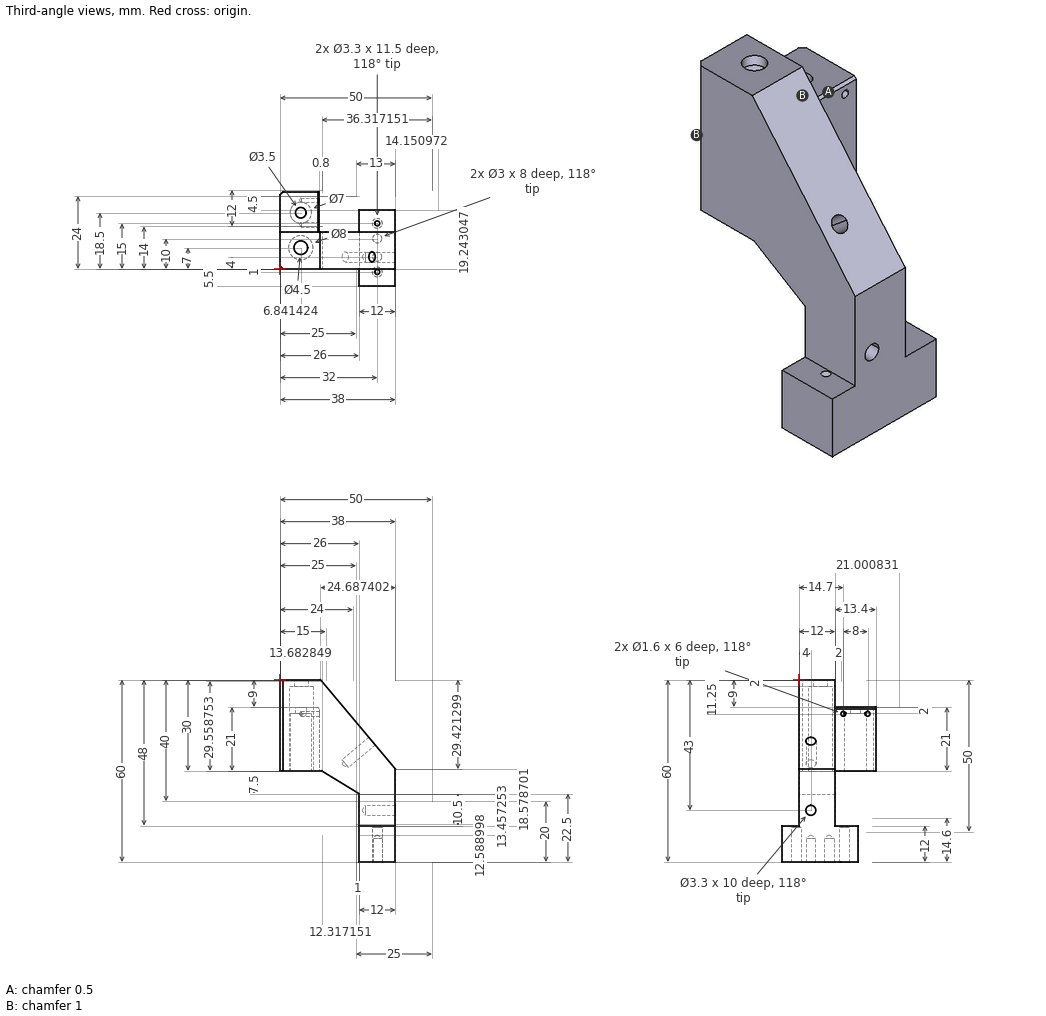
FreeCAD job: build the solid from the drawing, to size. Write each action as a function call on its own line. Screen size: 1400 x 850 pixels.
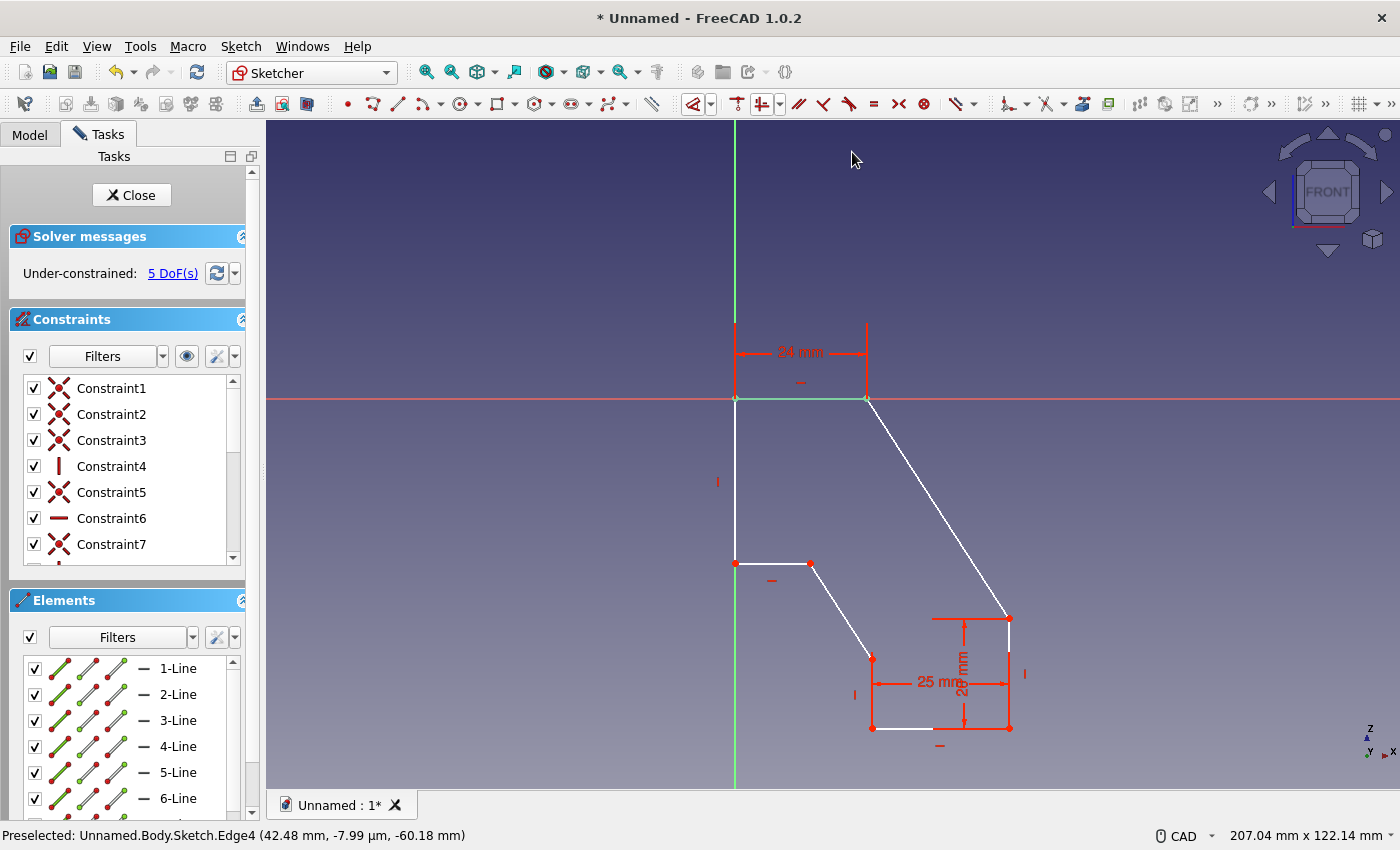
click(735, 514)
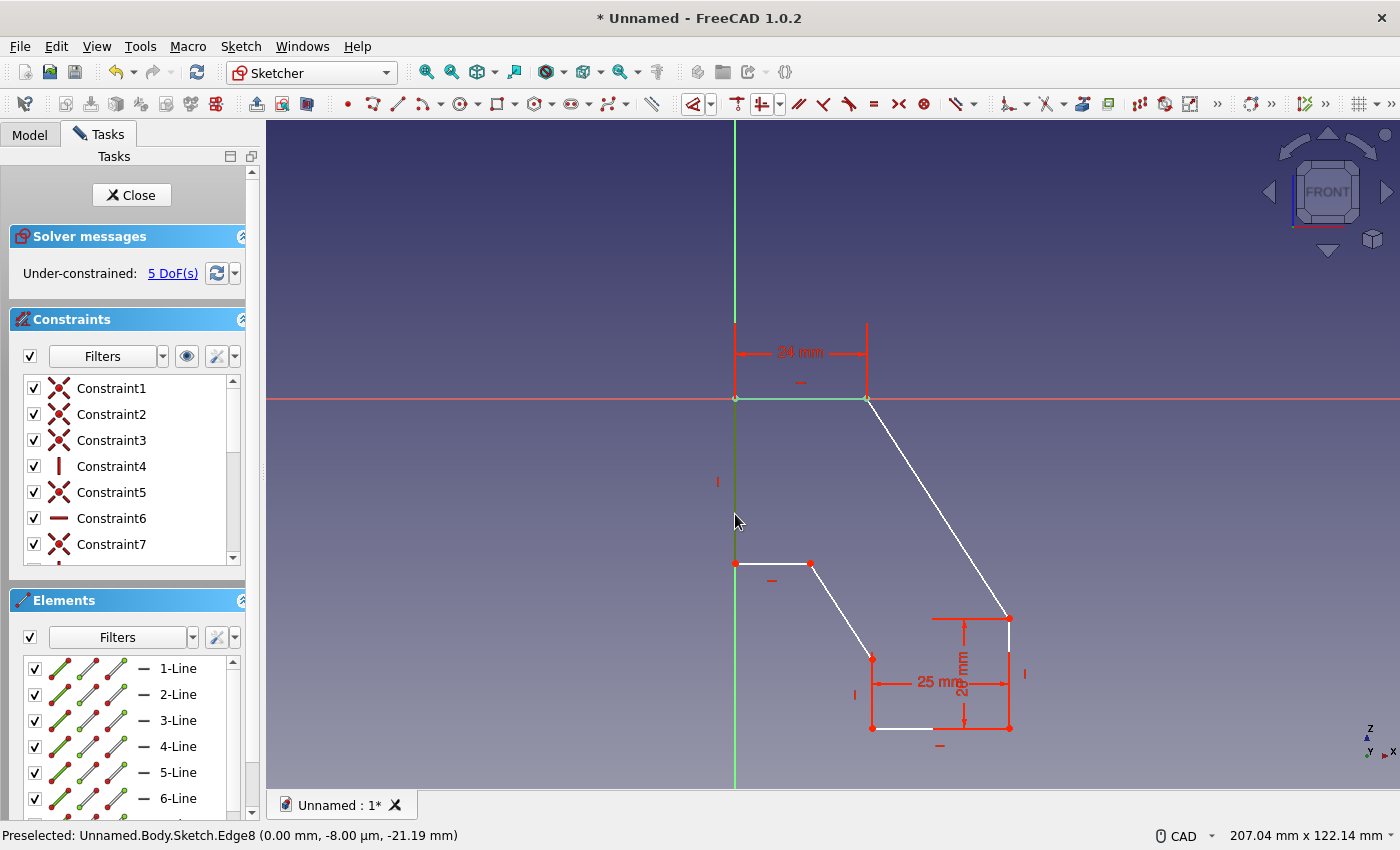
key(i)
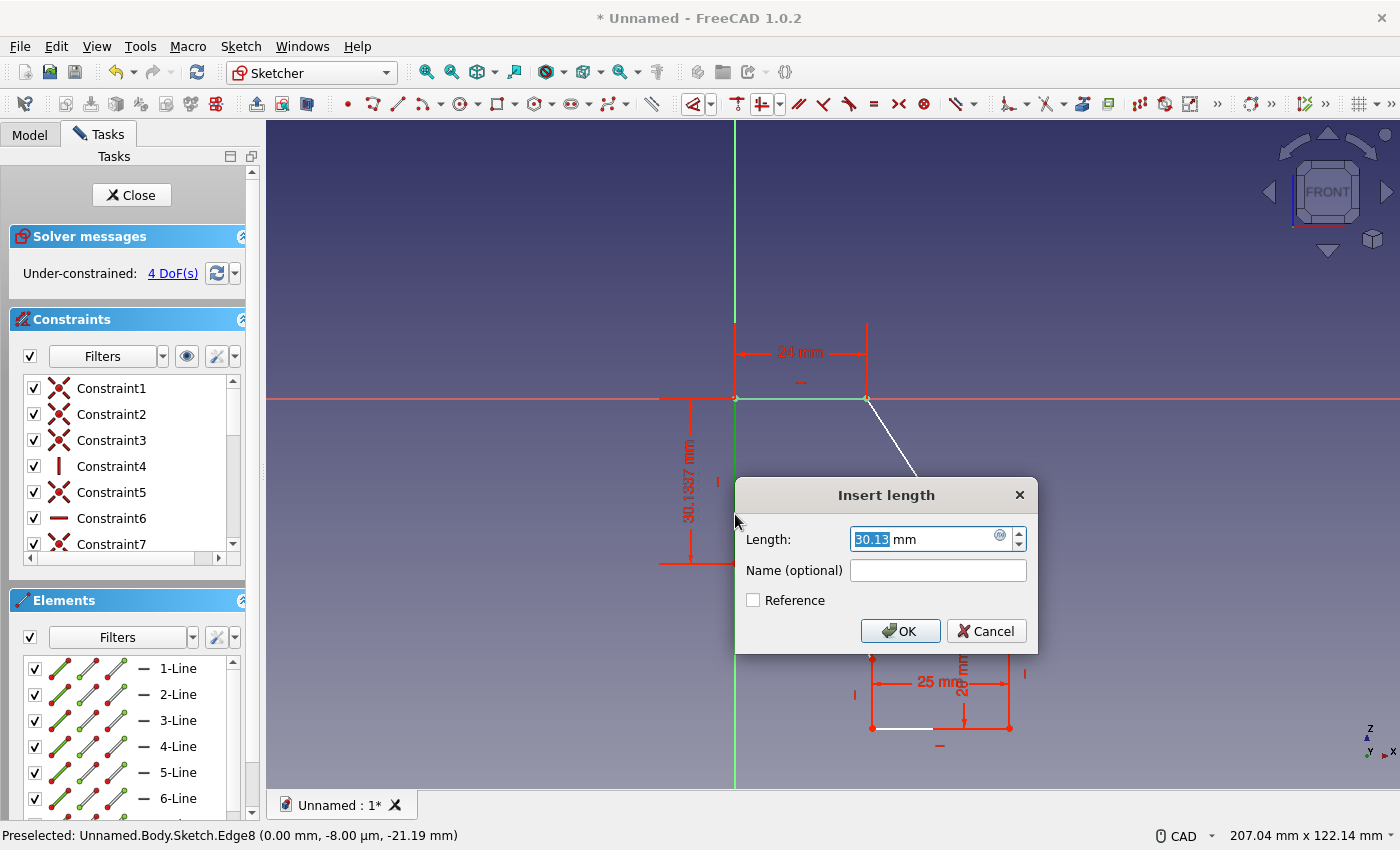
text(30)
key(Return)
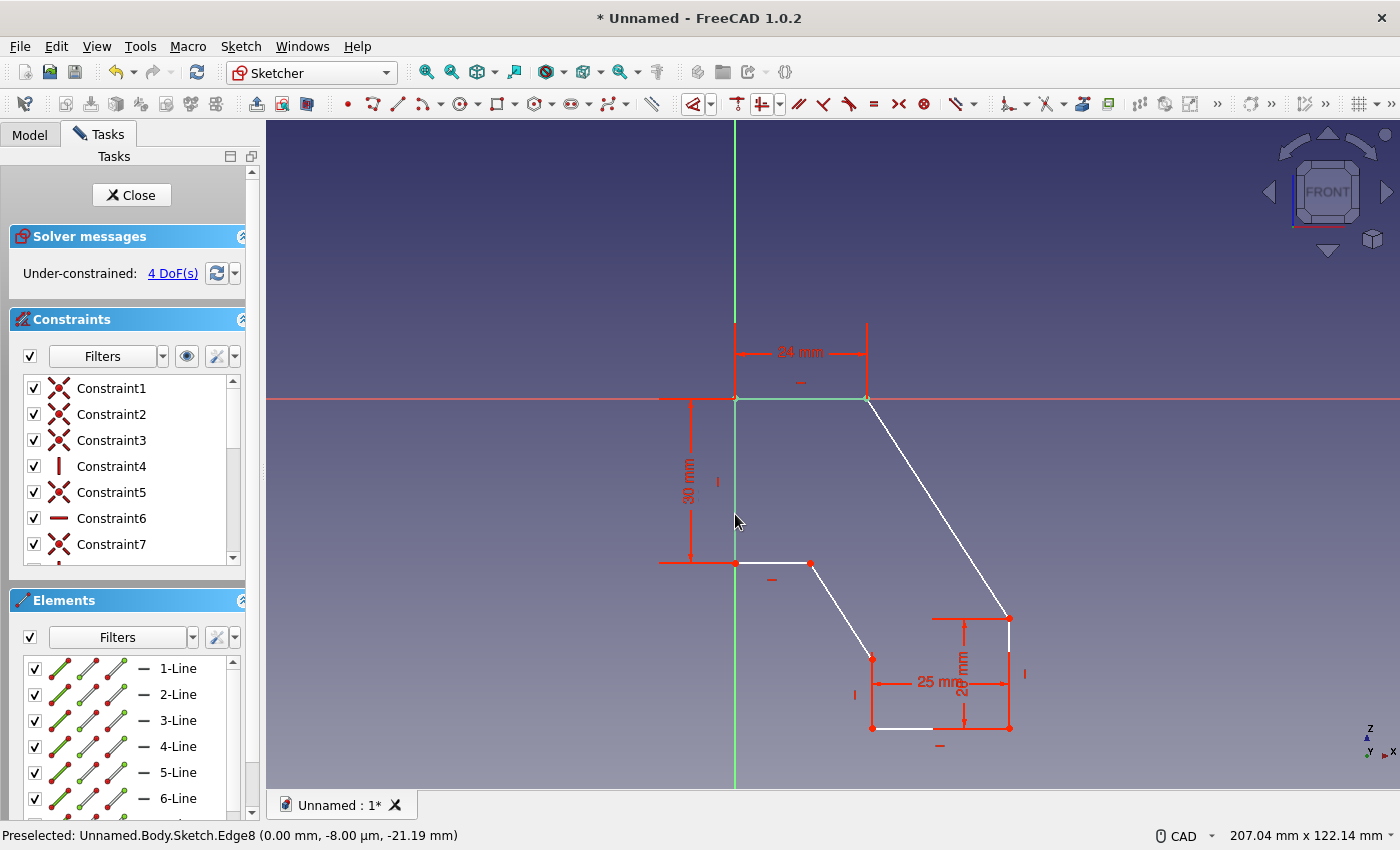
click(1009, 619)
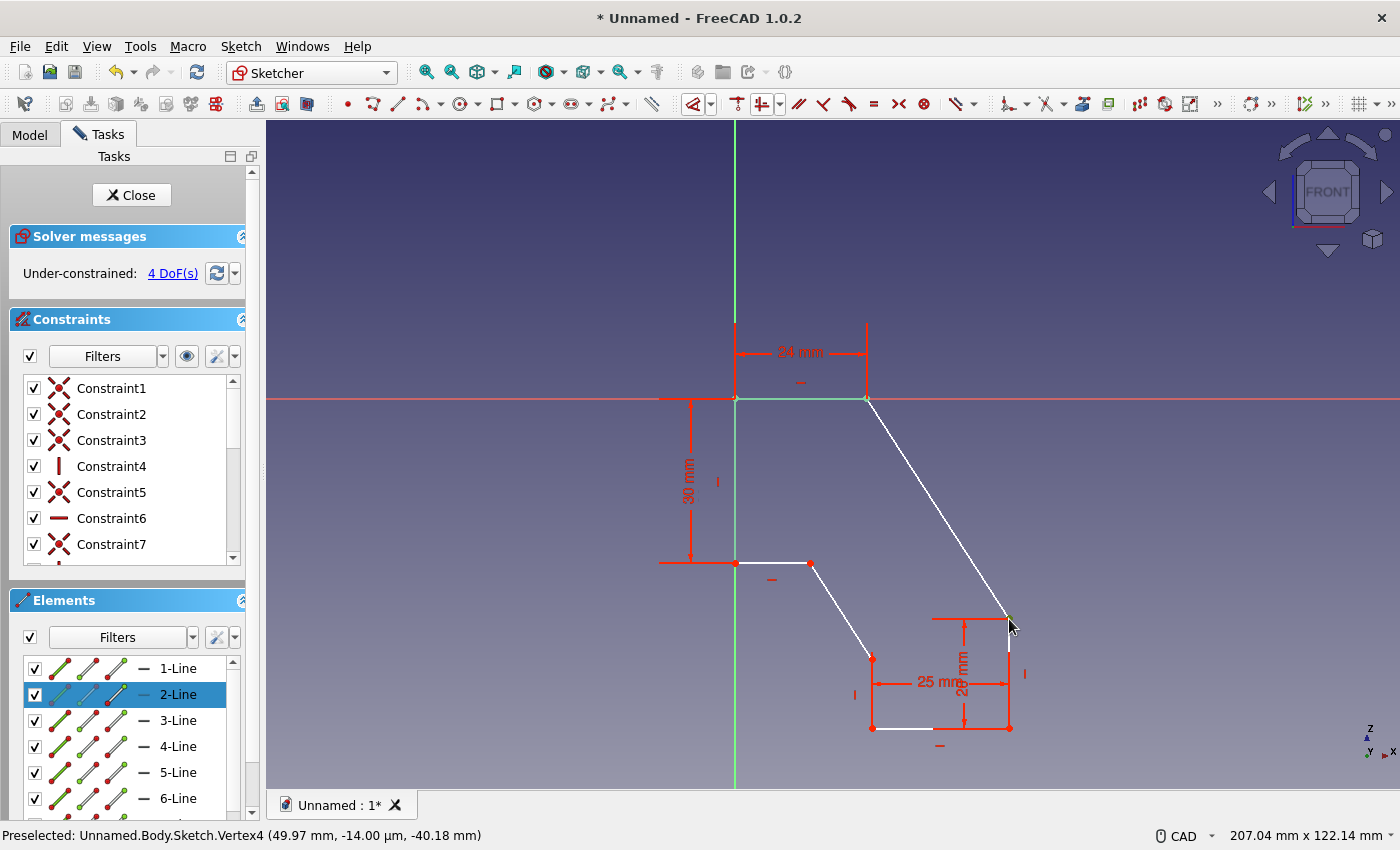
click(710, 104)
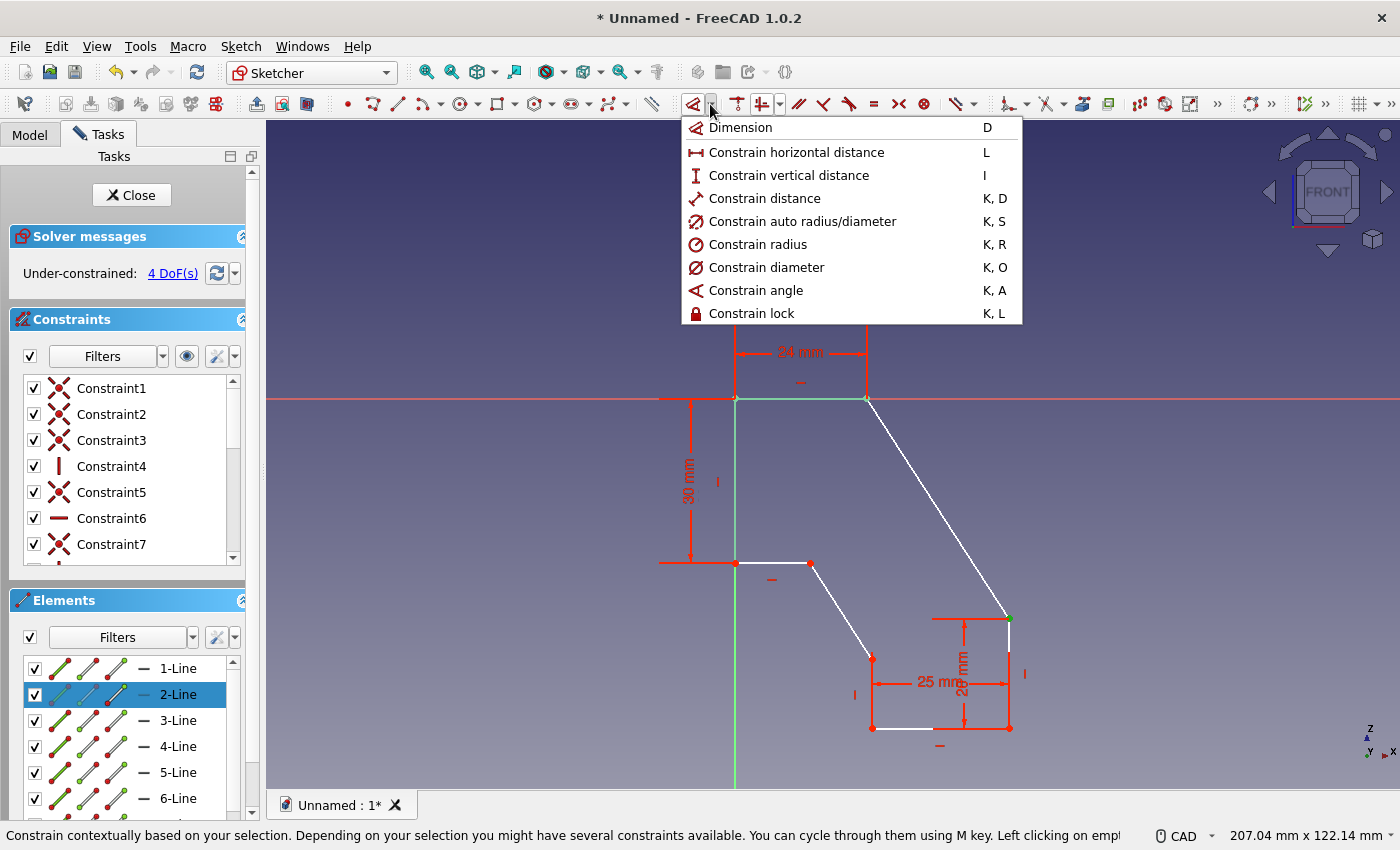
click(852, 152)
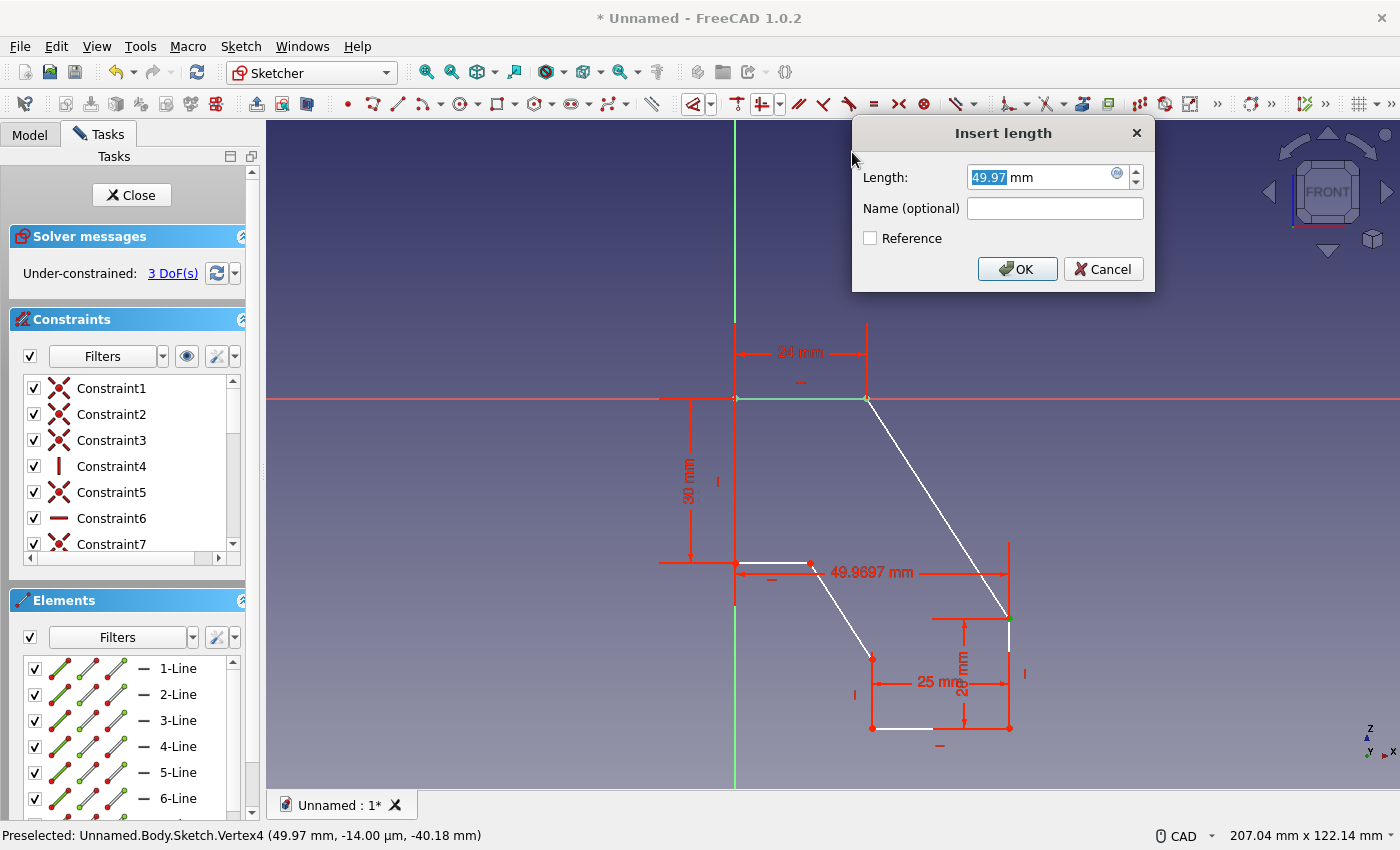
text(50)
key(Return)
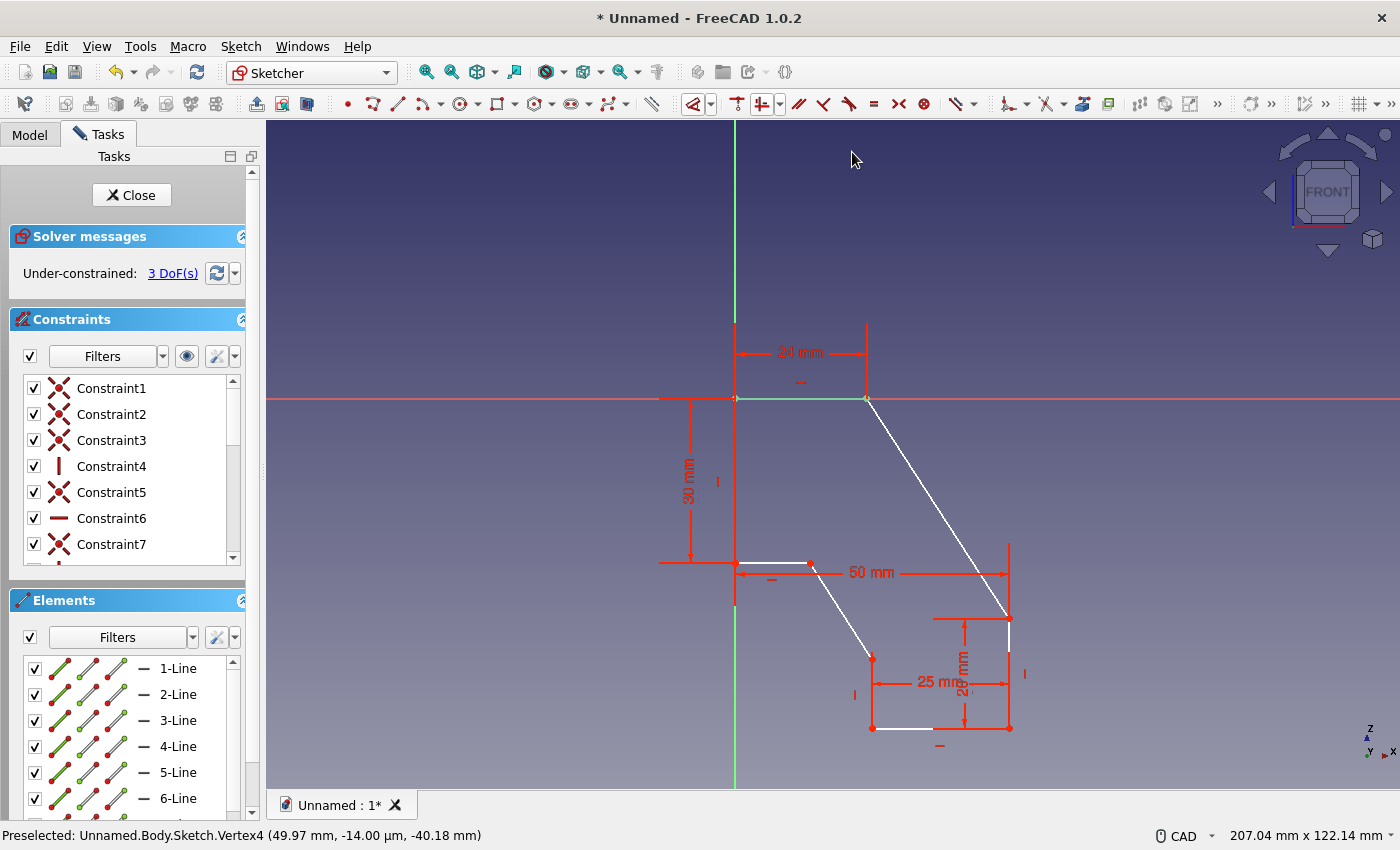
click(1009, 619)